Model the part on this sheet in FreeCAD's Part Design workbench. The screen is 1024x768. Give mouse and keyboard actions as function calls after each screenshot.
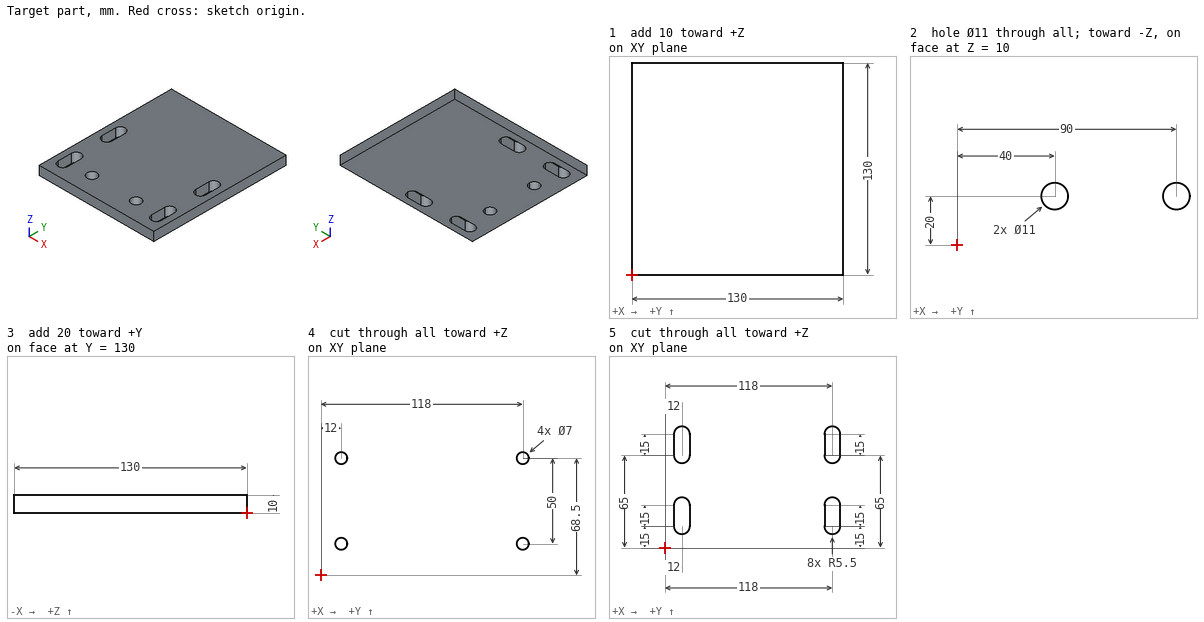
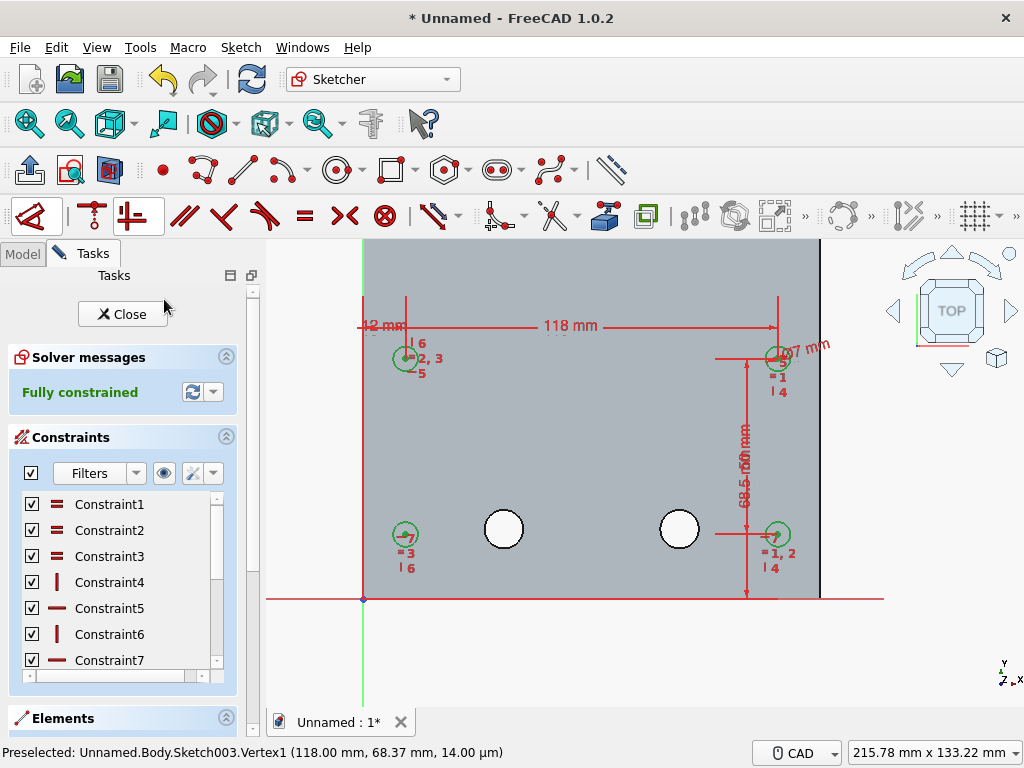
click(123, 314)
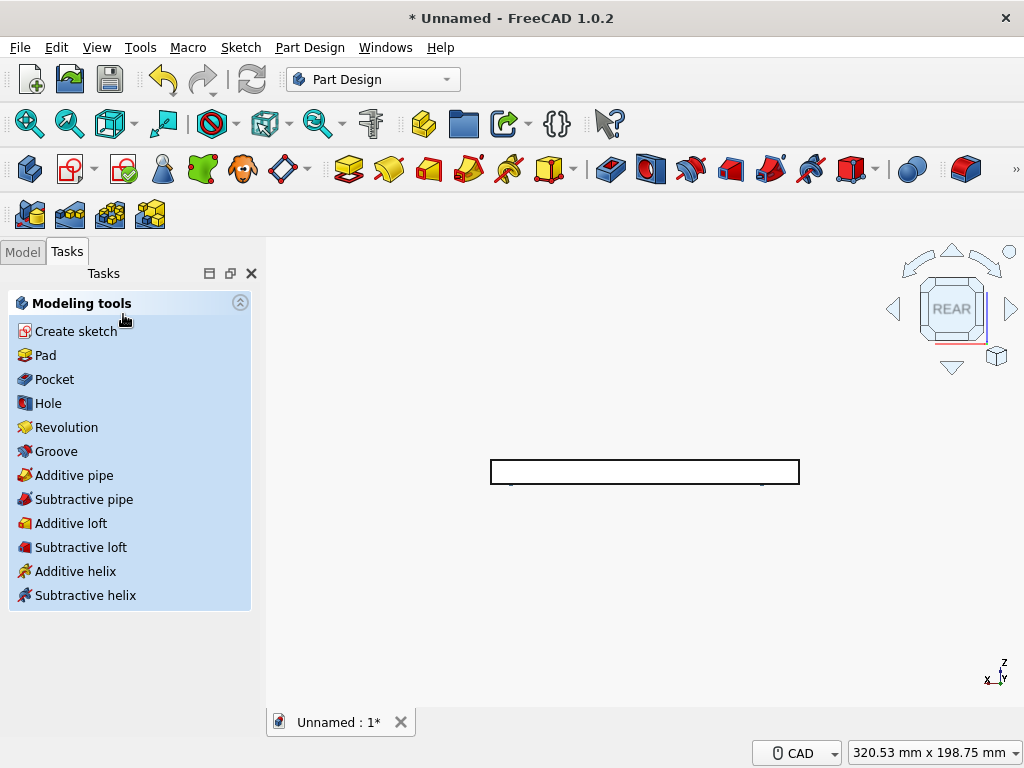
click(612, 170)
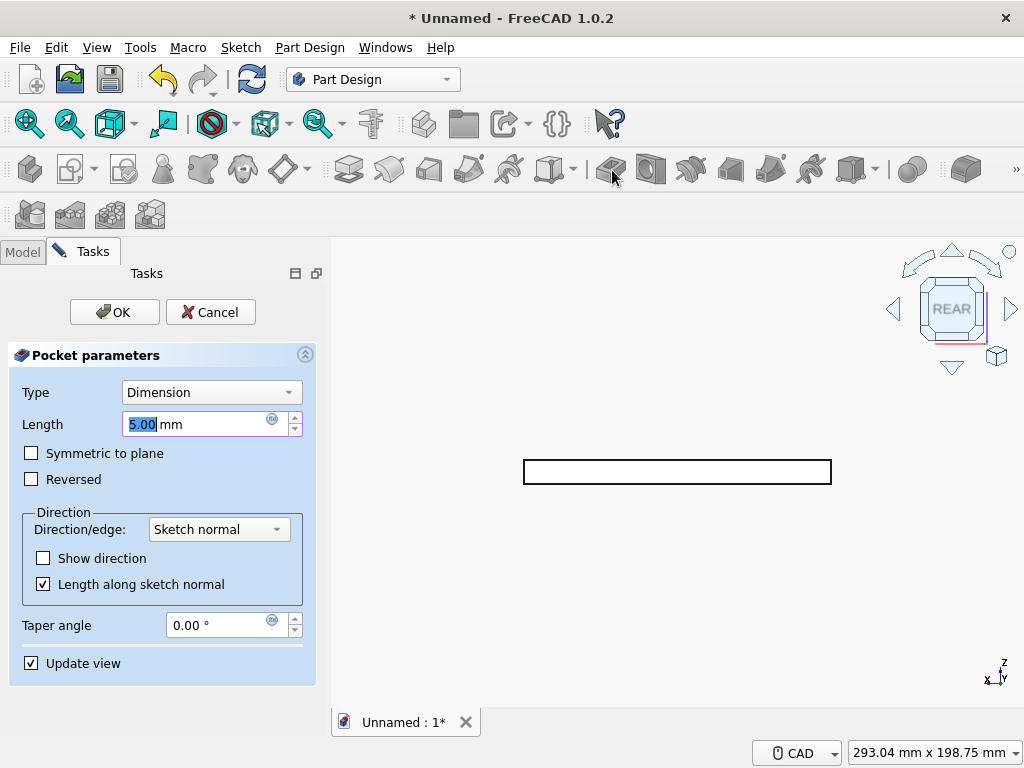
click(212, 392)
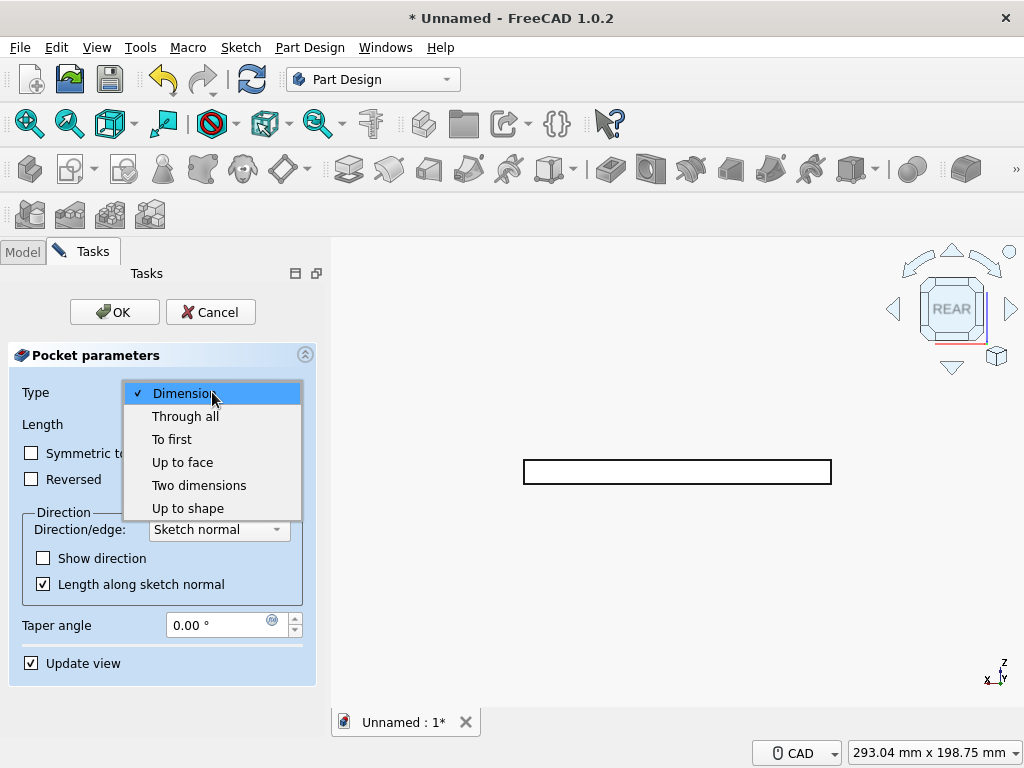
click(212, 416)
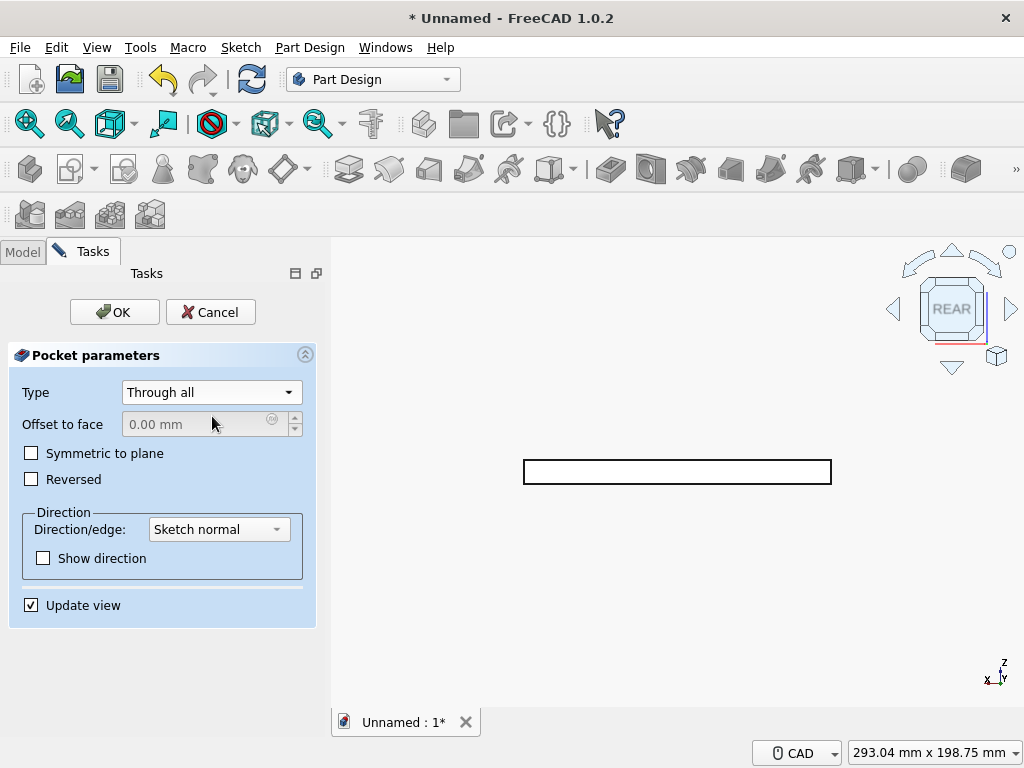
click(30, 479)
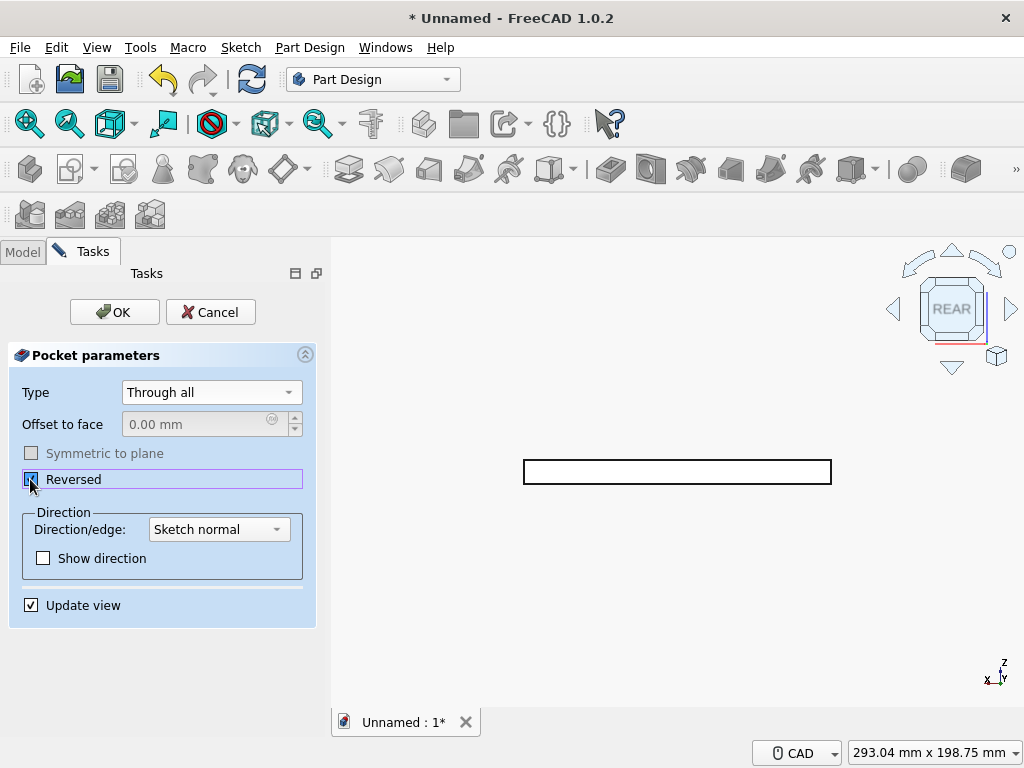
click(115, 312)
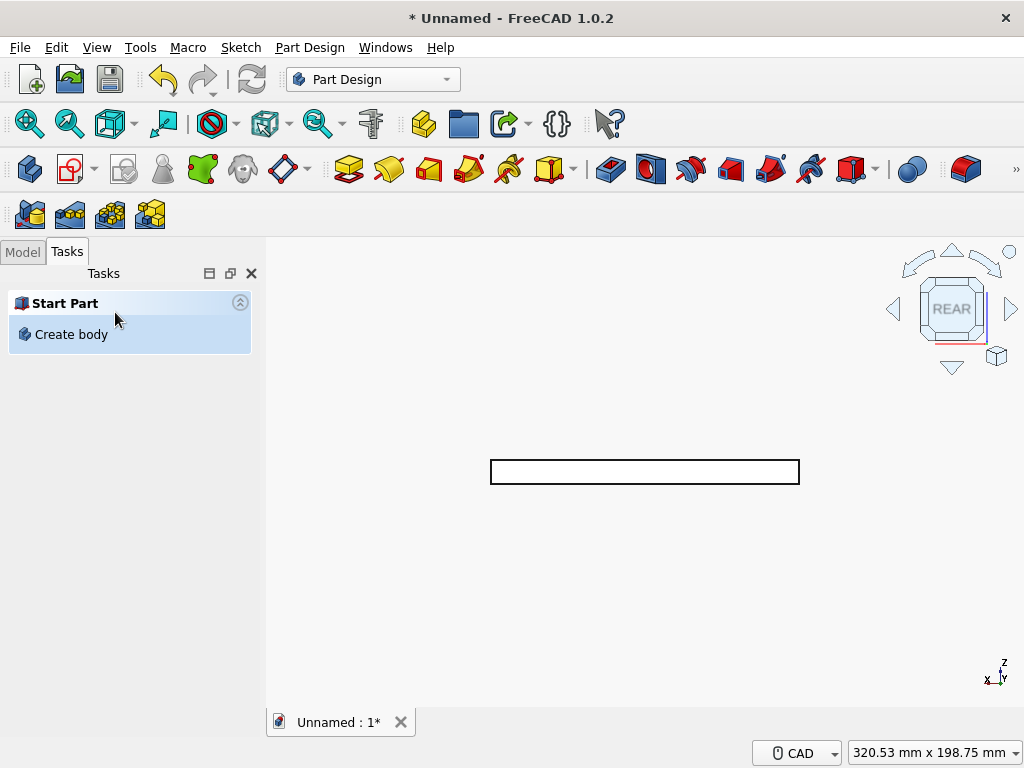
click(30, 124)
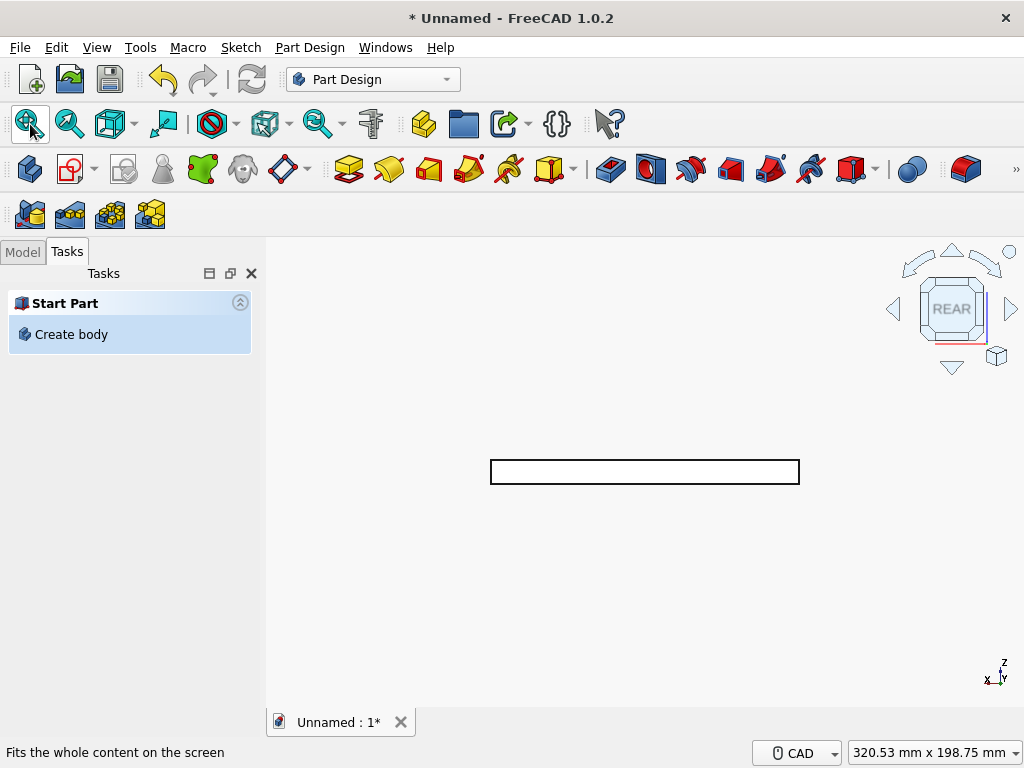
click(70, 170)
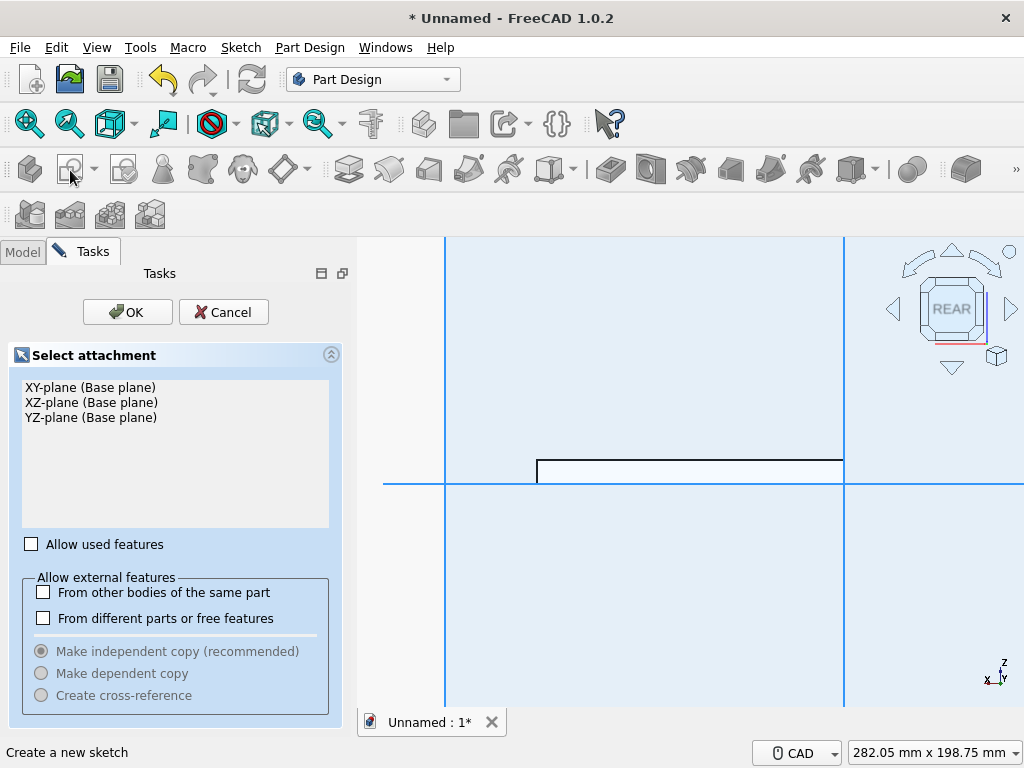
click(82, 388)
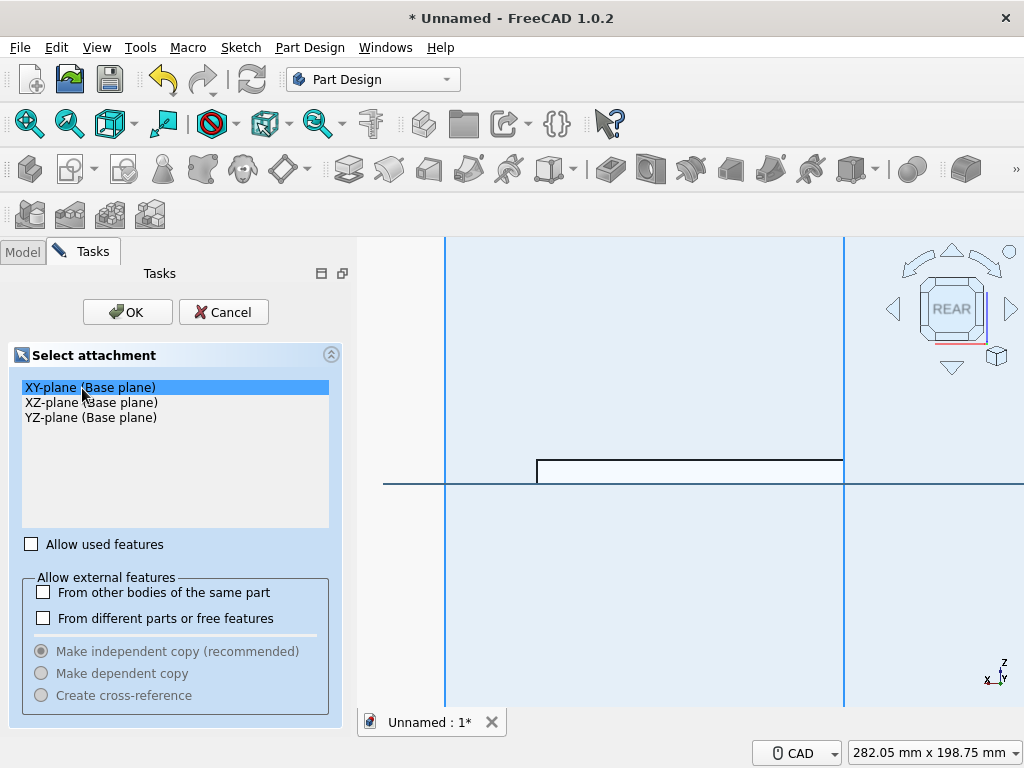
click(128, 312)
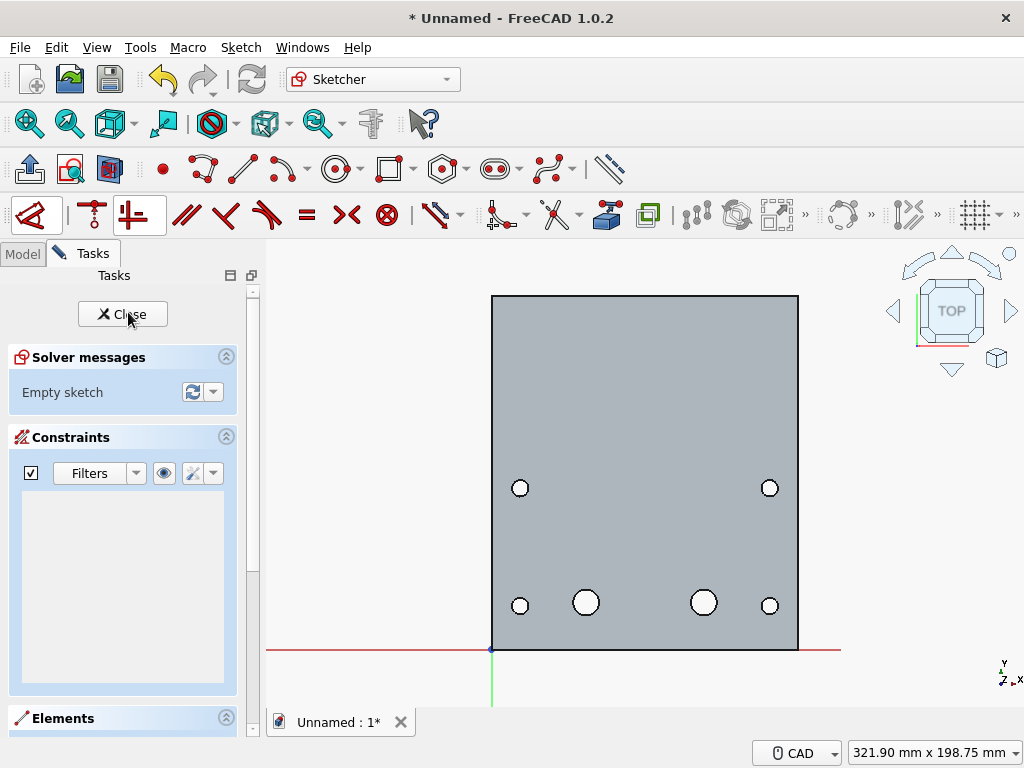
click(110, 170)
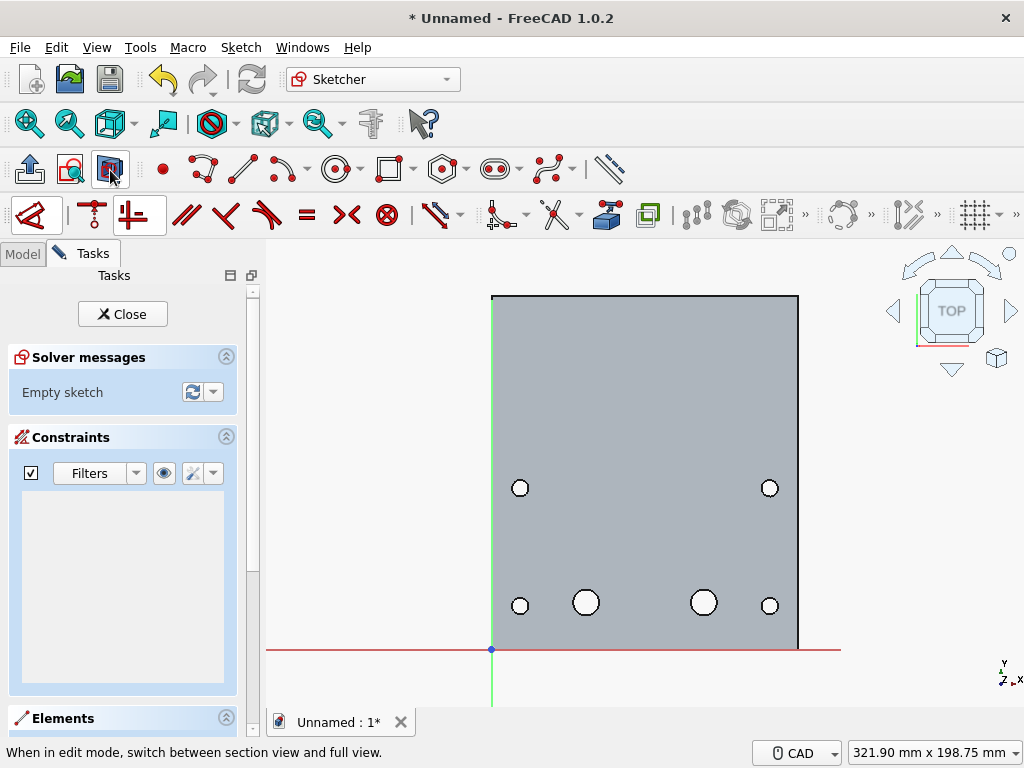
scroll(761, 679, up, 2)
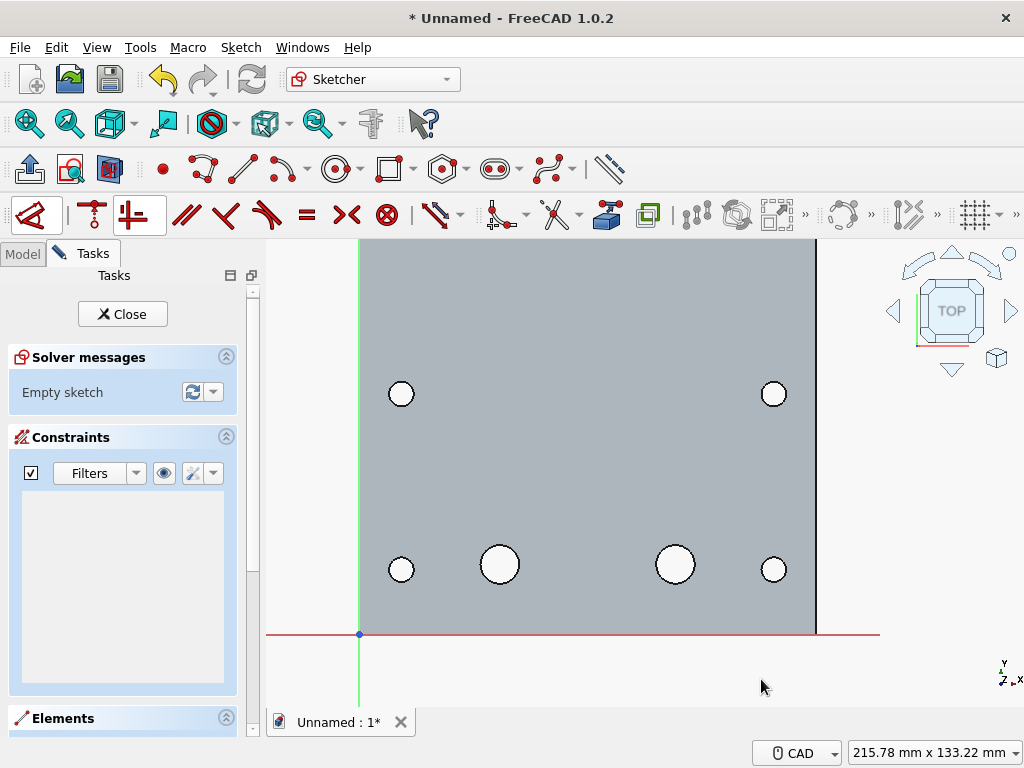
click(496, 170)